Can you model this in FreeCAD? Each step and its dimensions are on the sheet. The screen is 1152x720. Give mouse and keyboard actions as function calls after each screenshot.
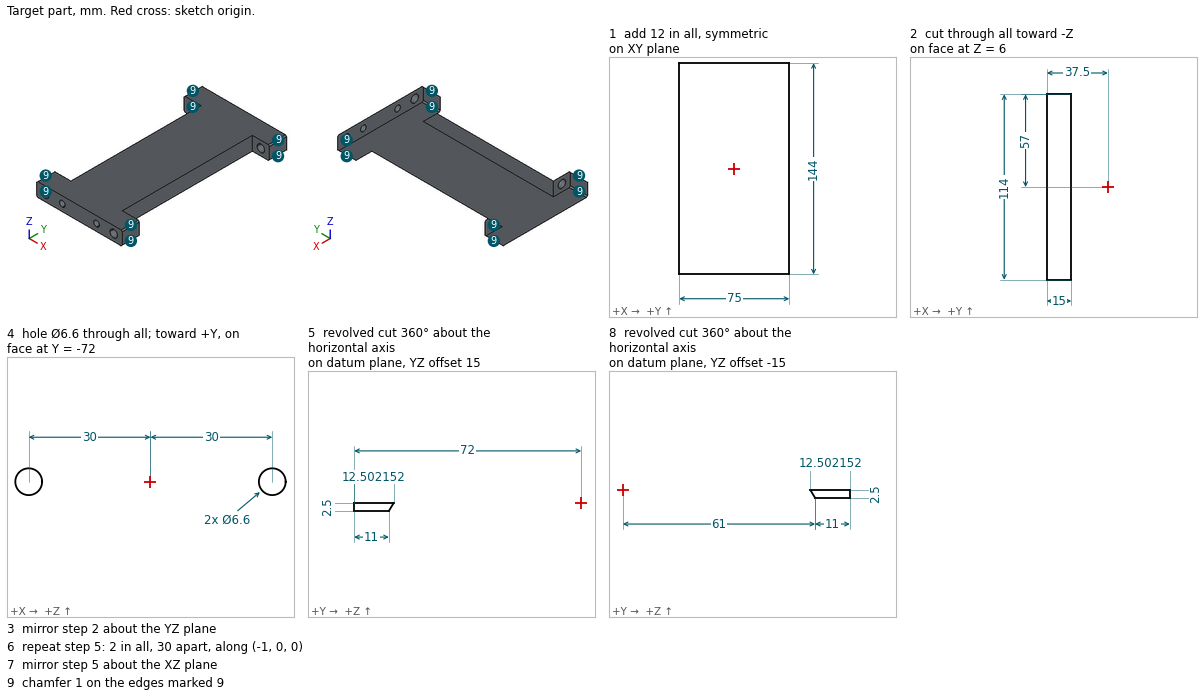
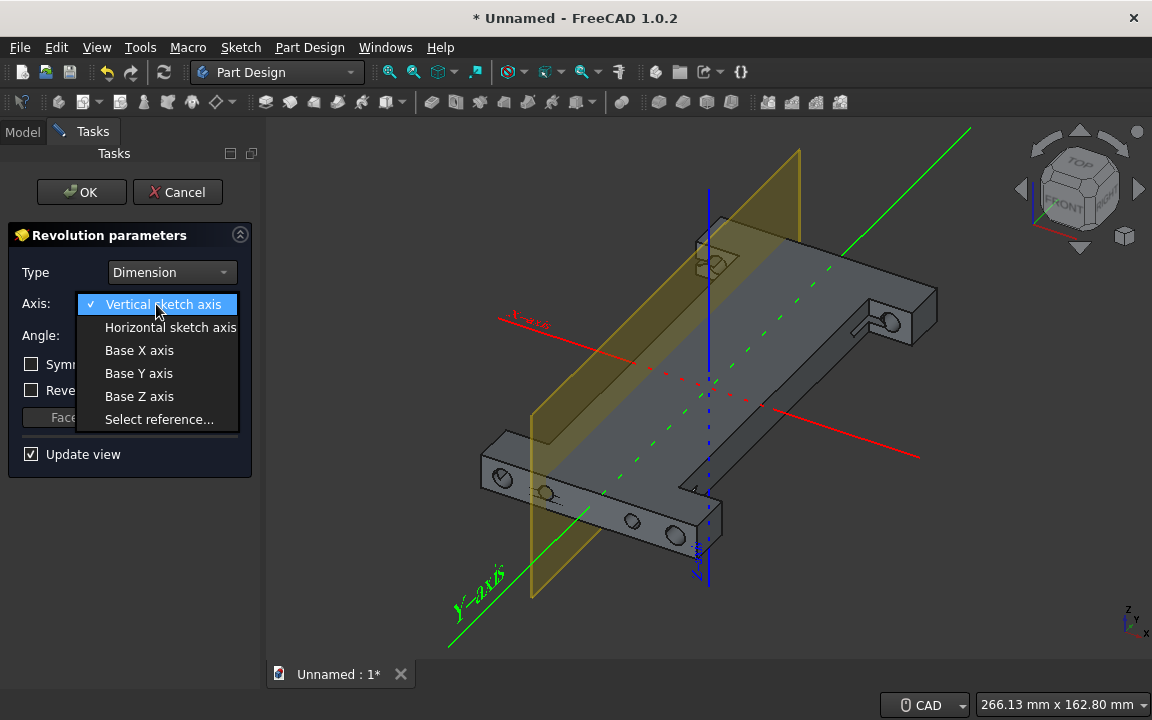
click(156, 328)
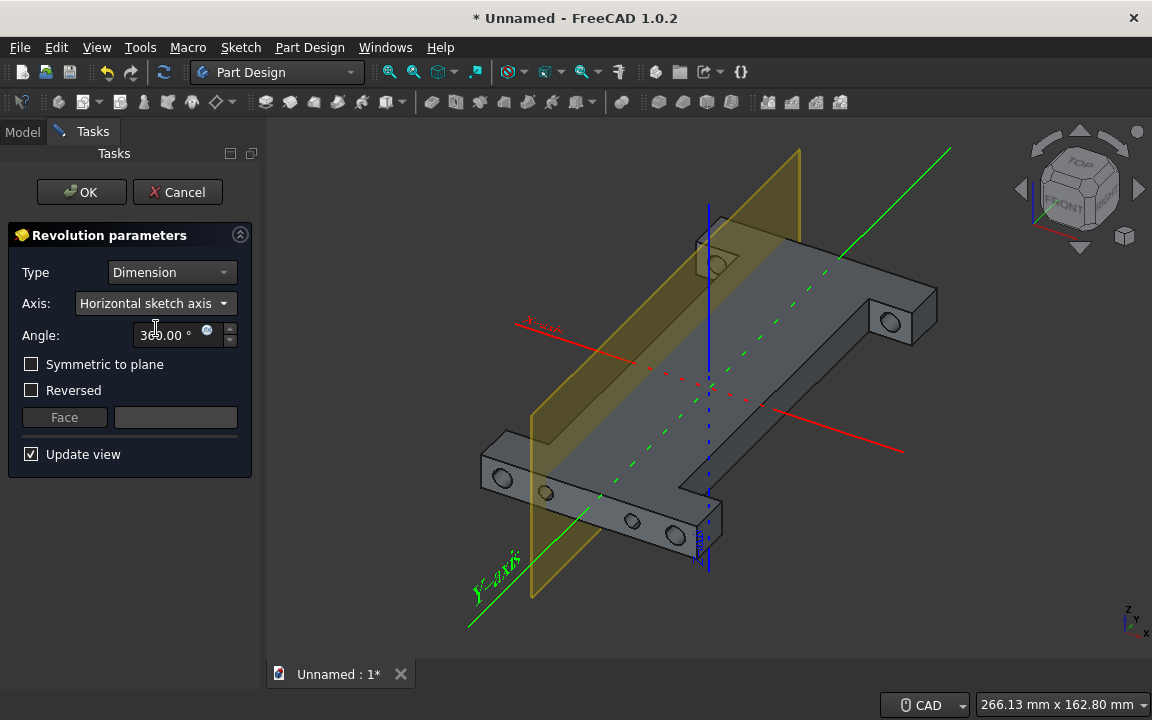
click(82, 192)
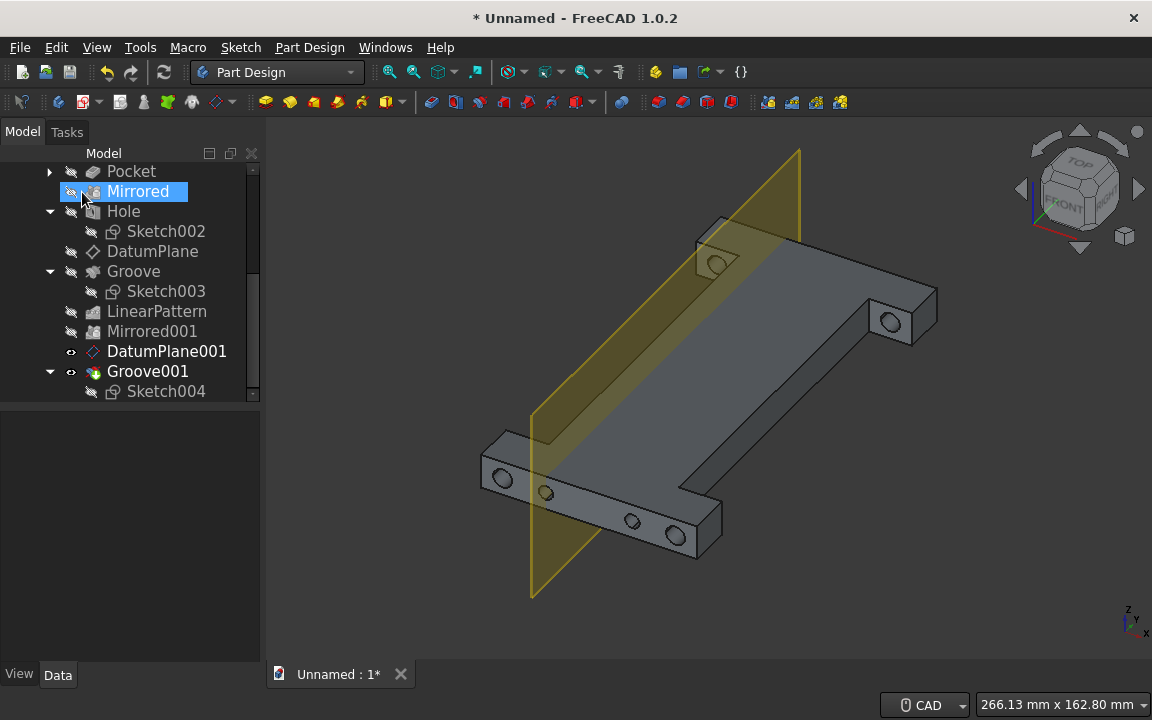
click(116, 352)
key(space)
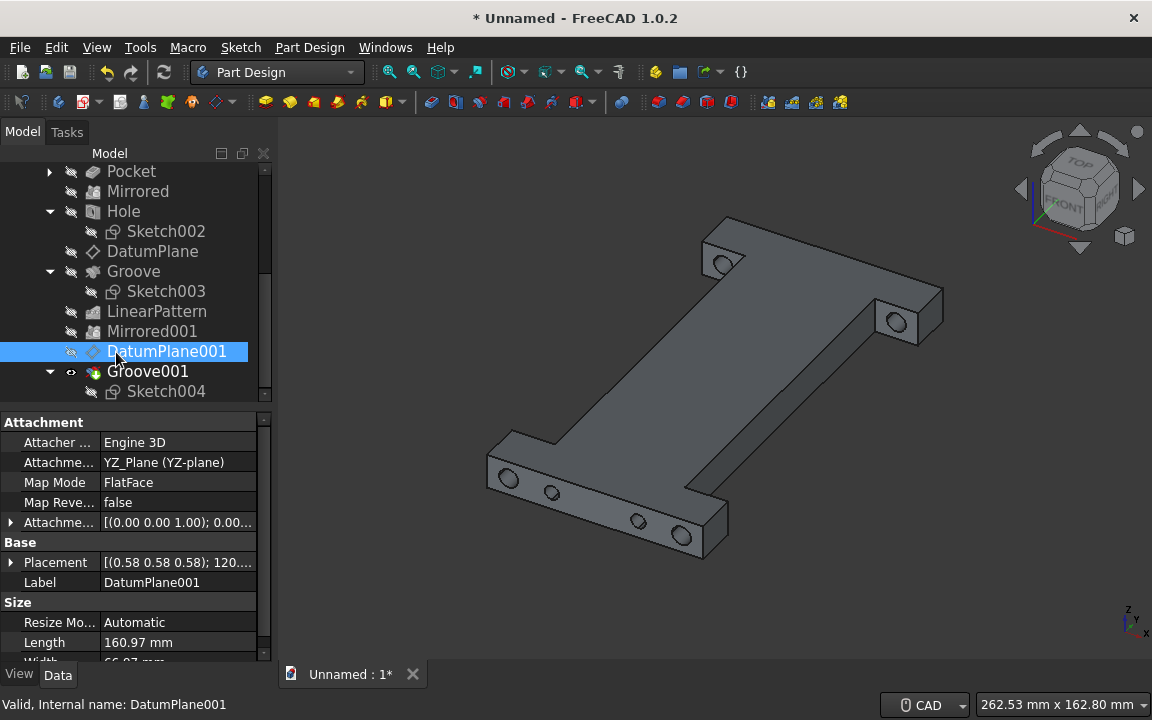
click(930, 300)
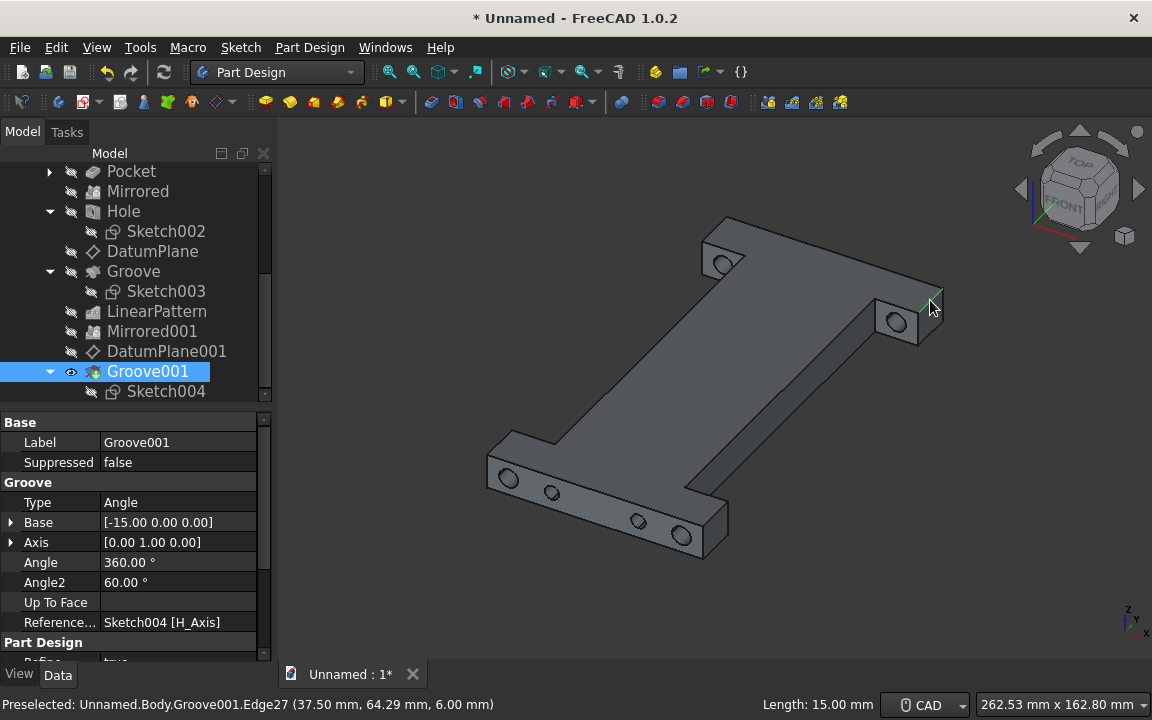
click(716, 513, ctrl)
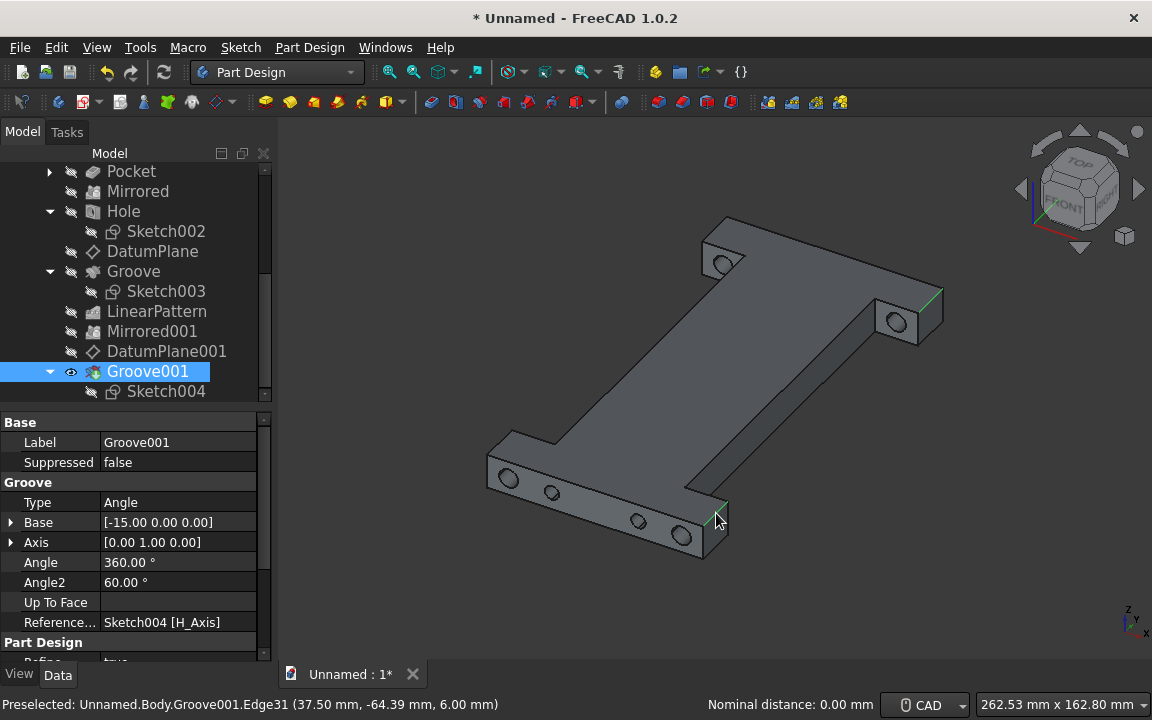
key(0)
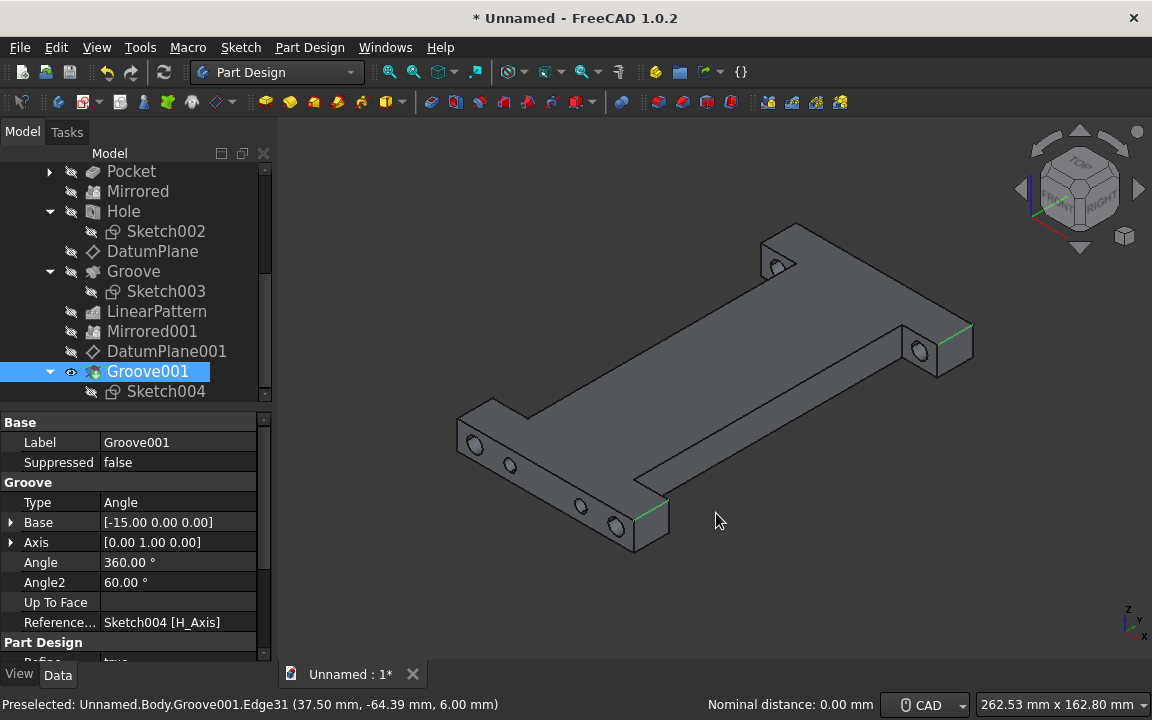
key(2)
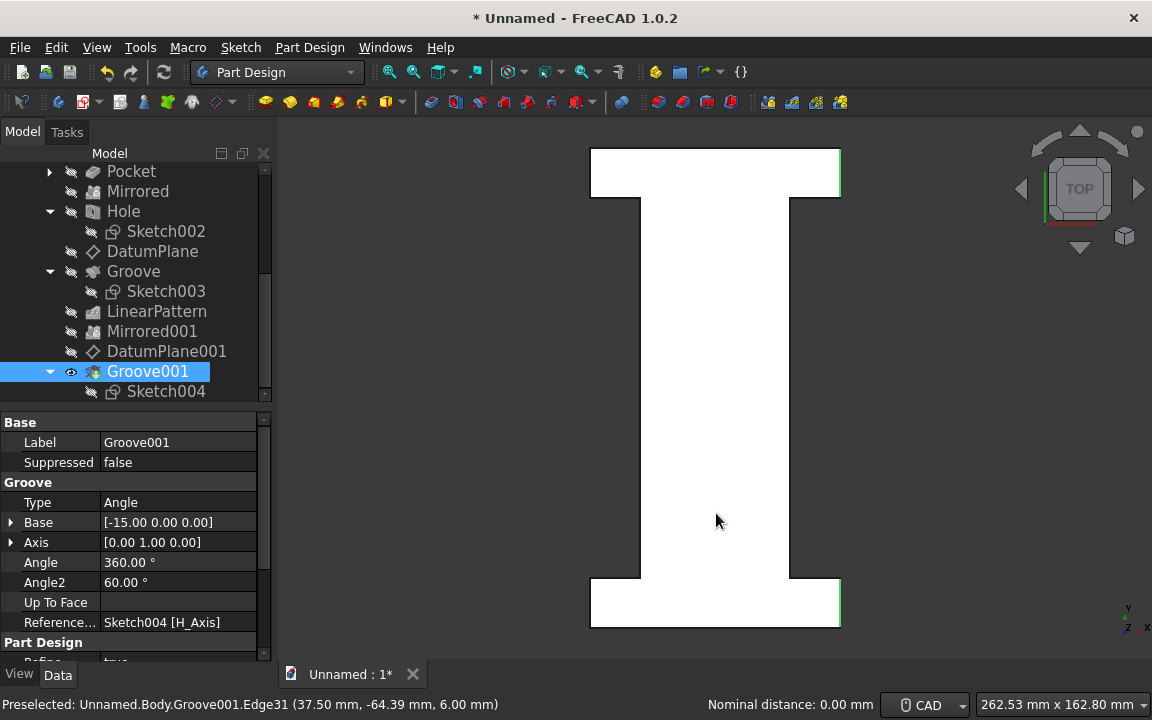
click(590, 172, ctrl)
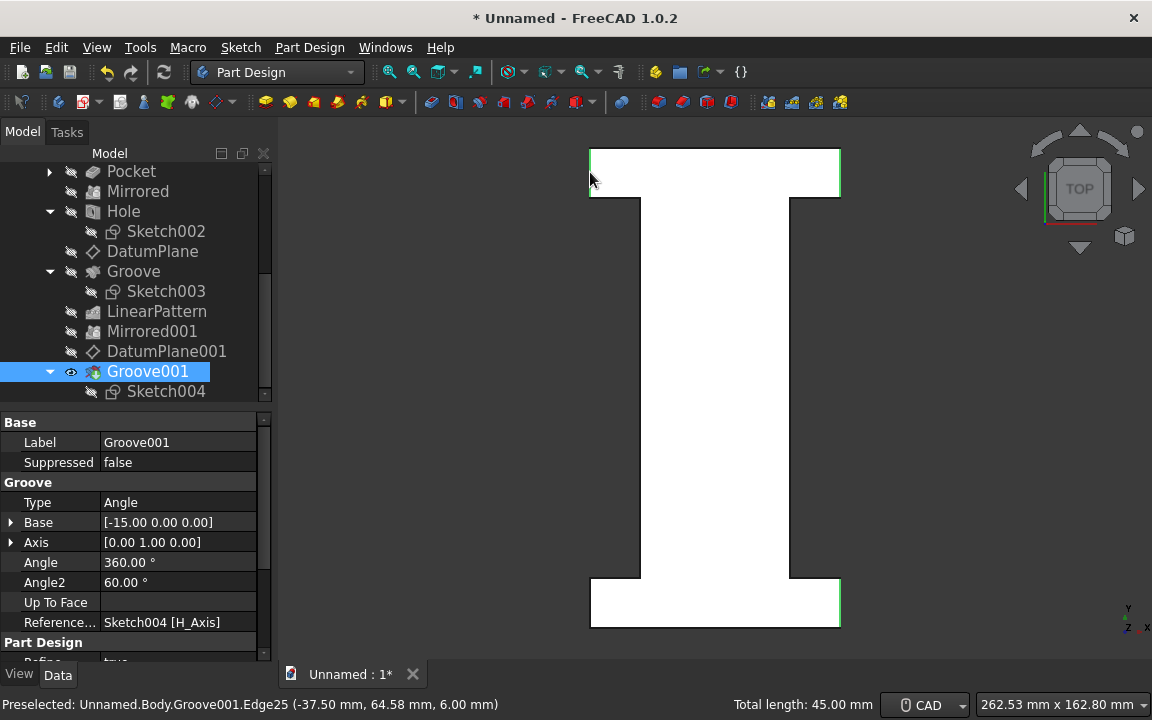
click(590, 602, ctrl)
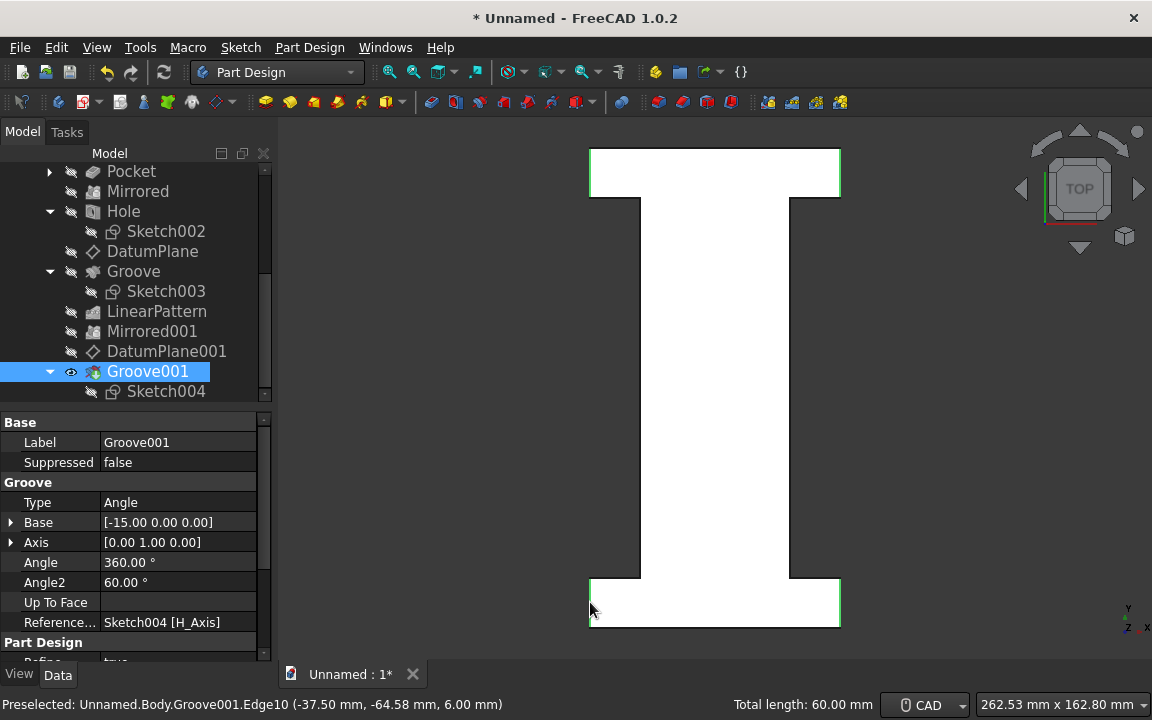
key(1)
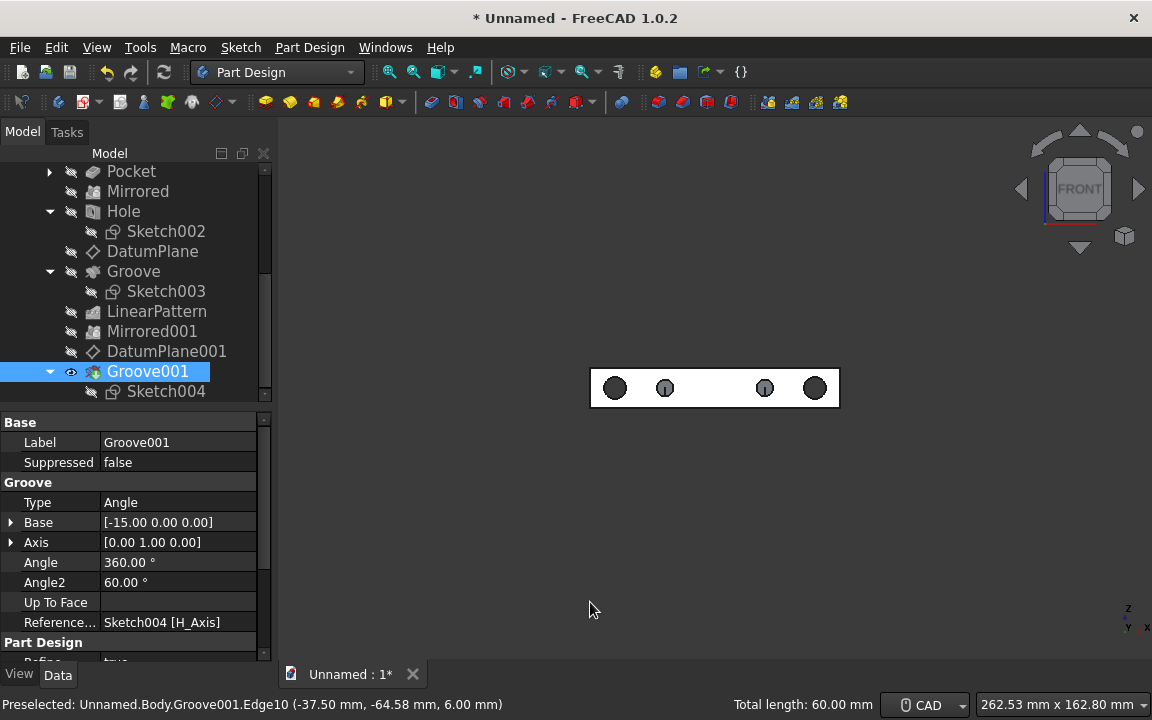
key(v)
key(f)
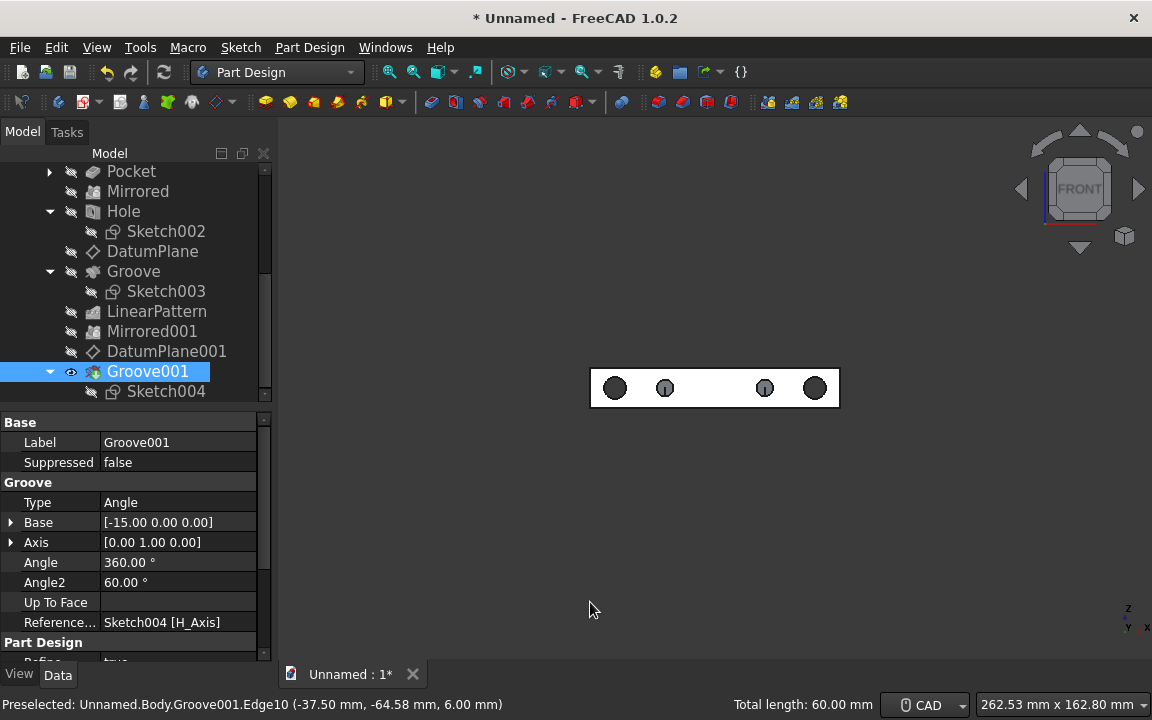
key(3)